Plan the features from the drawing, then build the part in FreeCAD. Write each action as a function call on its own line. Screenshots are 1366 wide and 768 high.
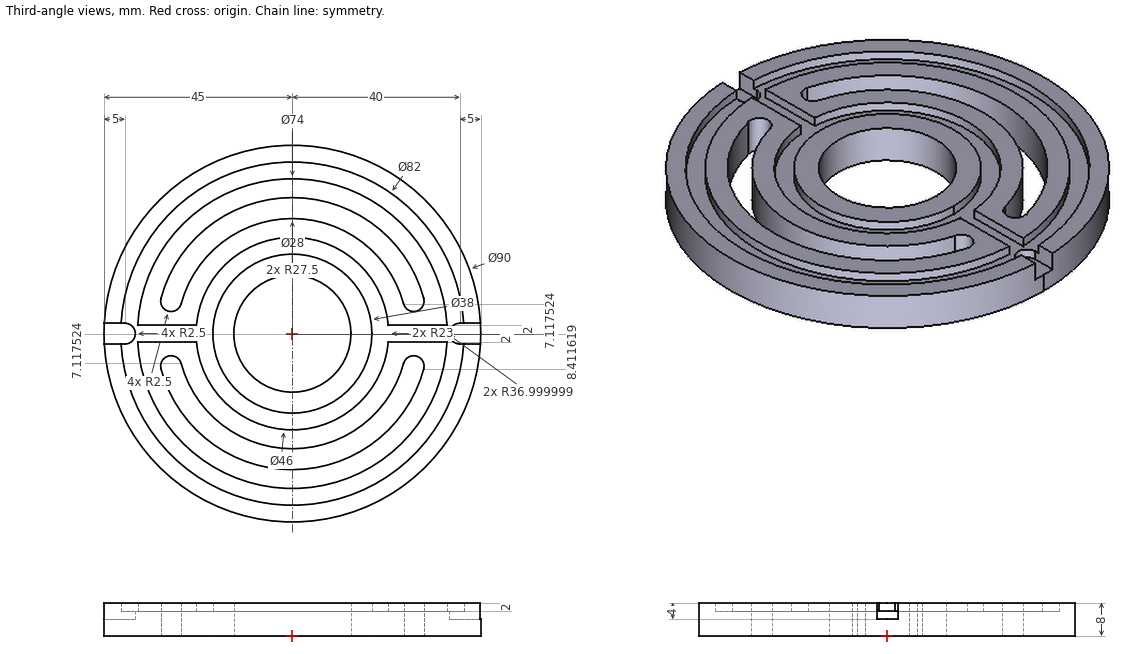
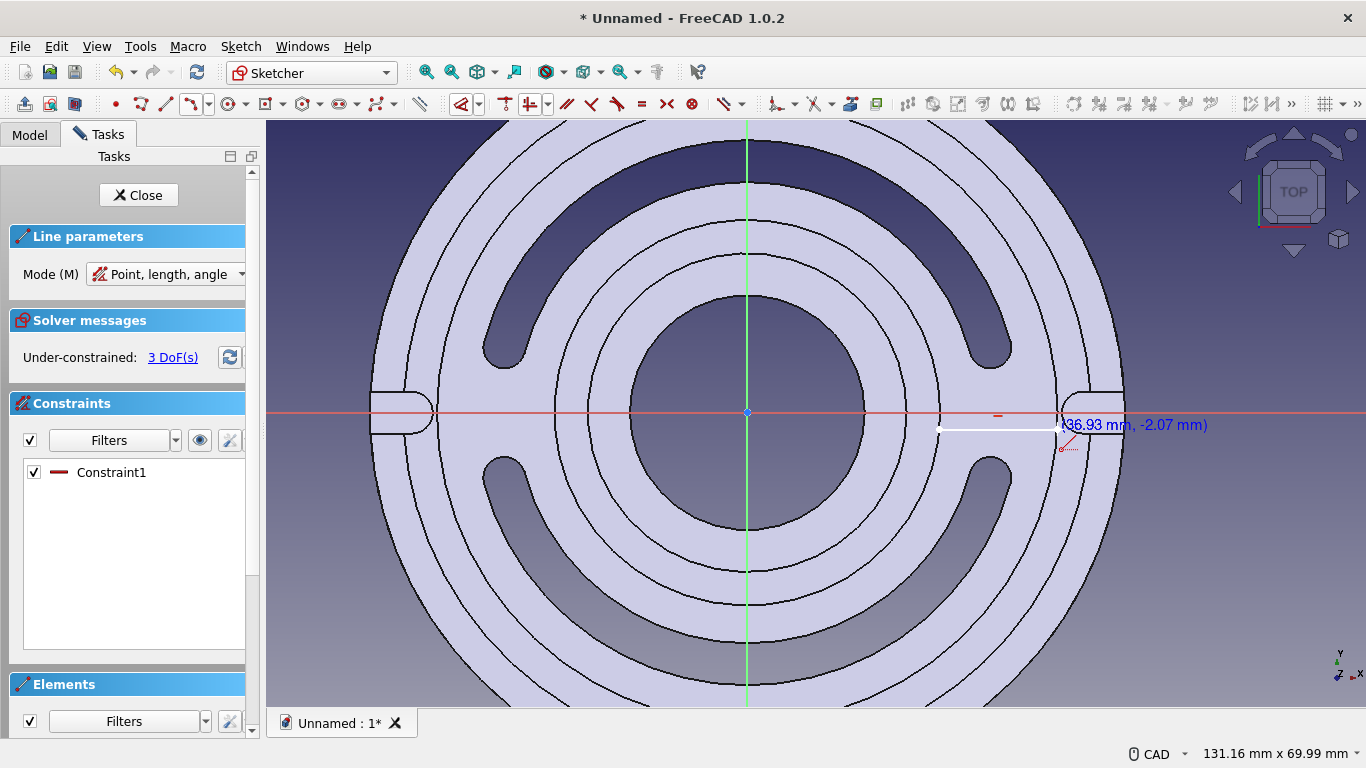
click(1057, 396)
click(939, 396)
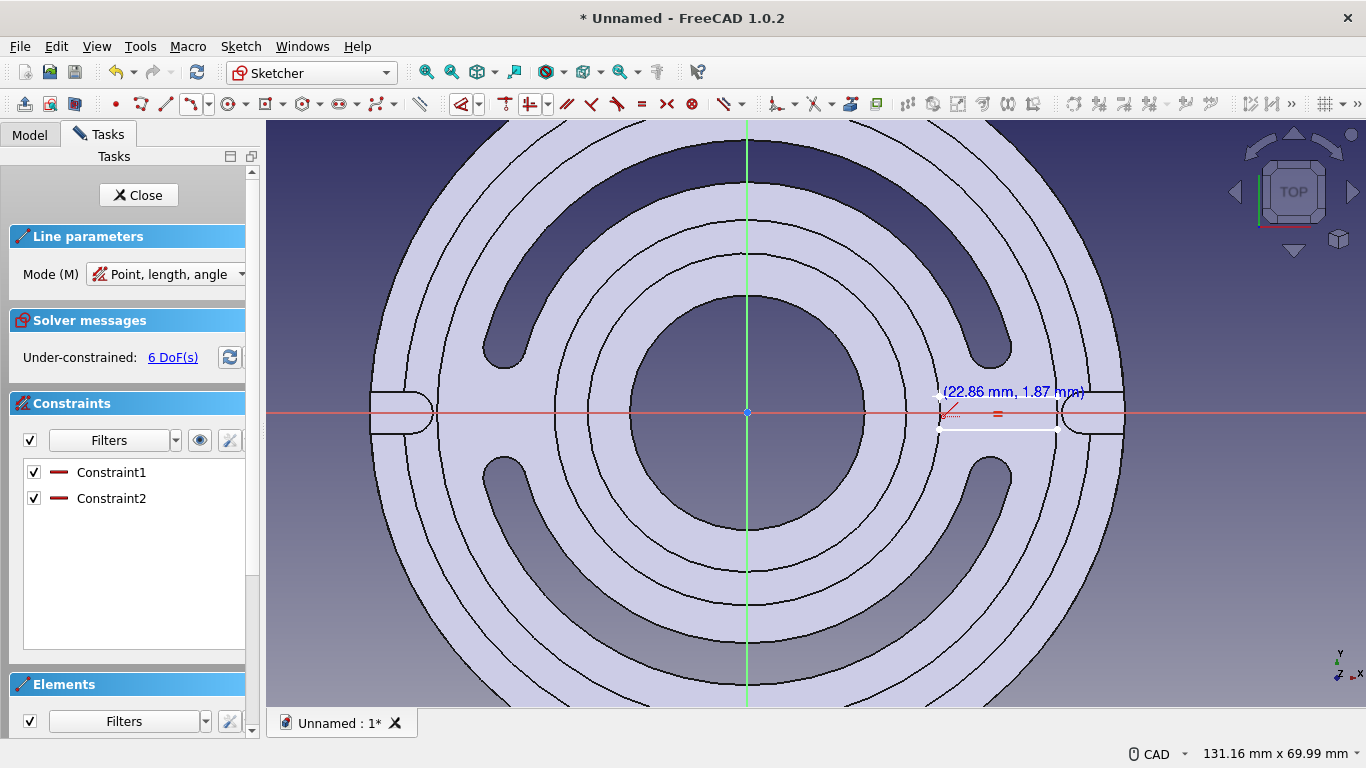
key(g)
key(3)
key(a)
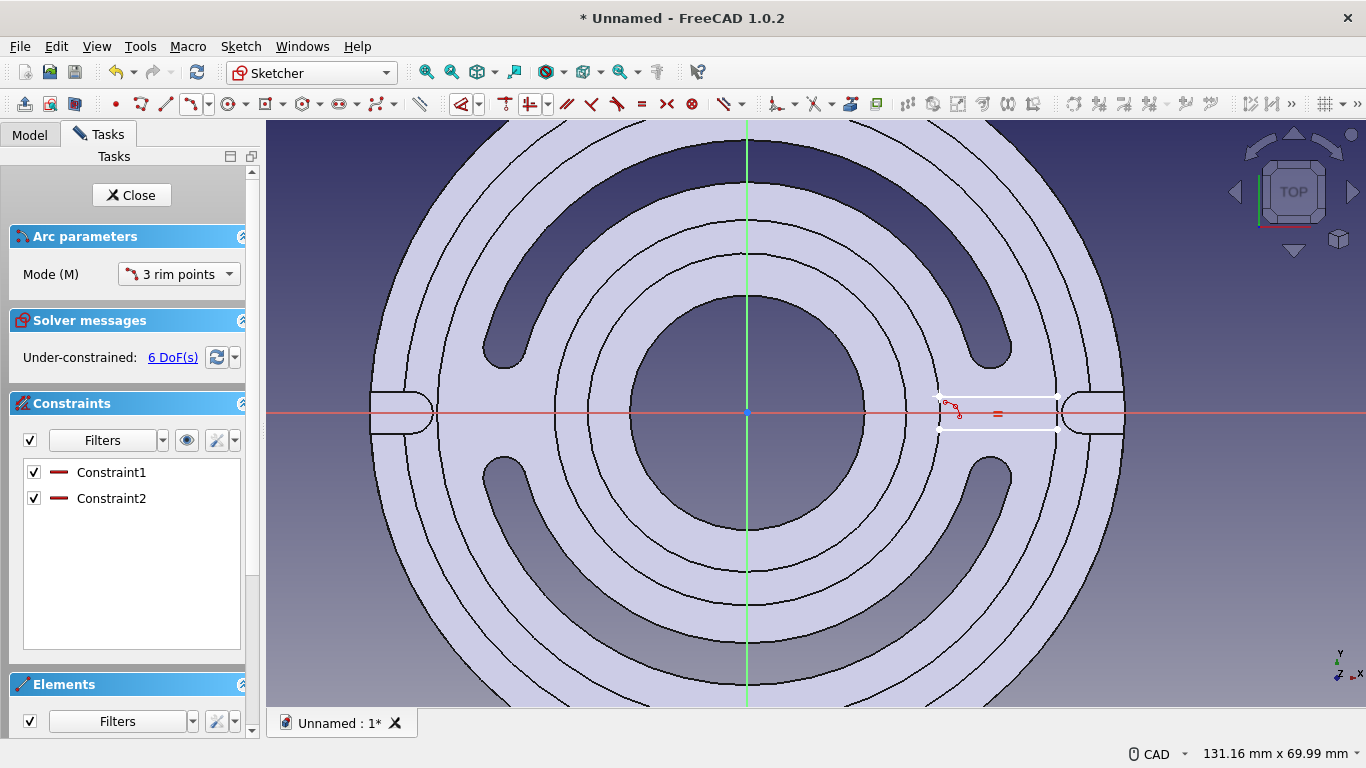
click(1057, 430)
click(1057, 397)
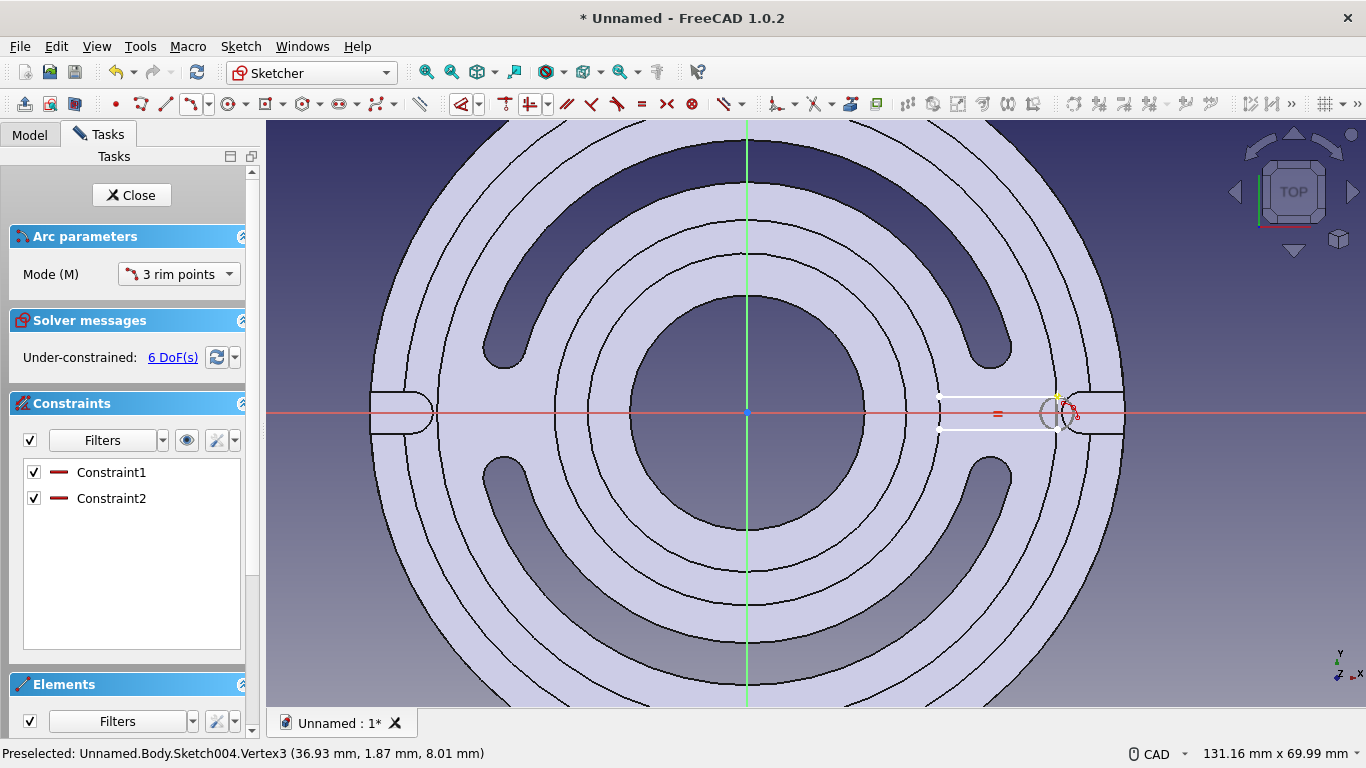
scroll(1058, 416, up, 18)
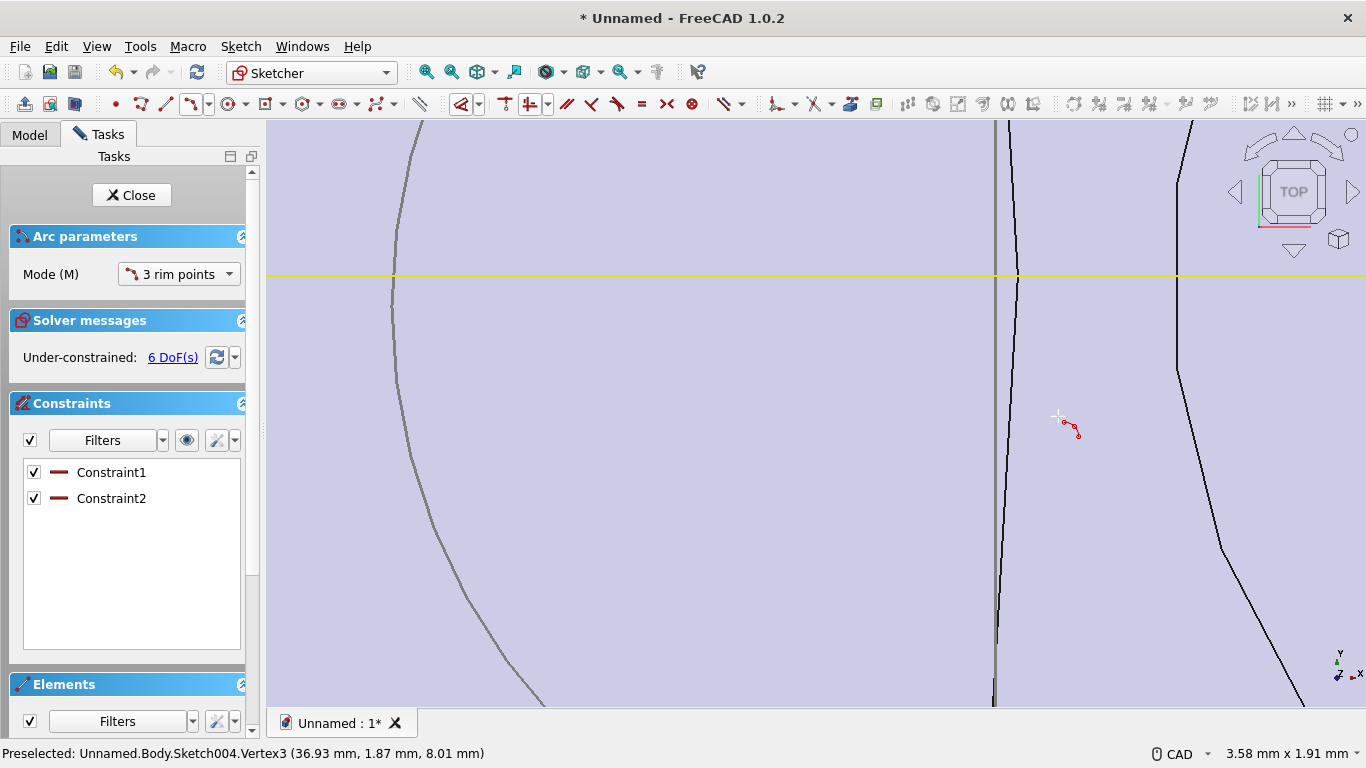
click(1017, 399)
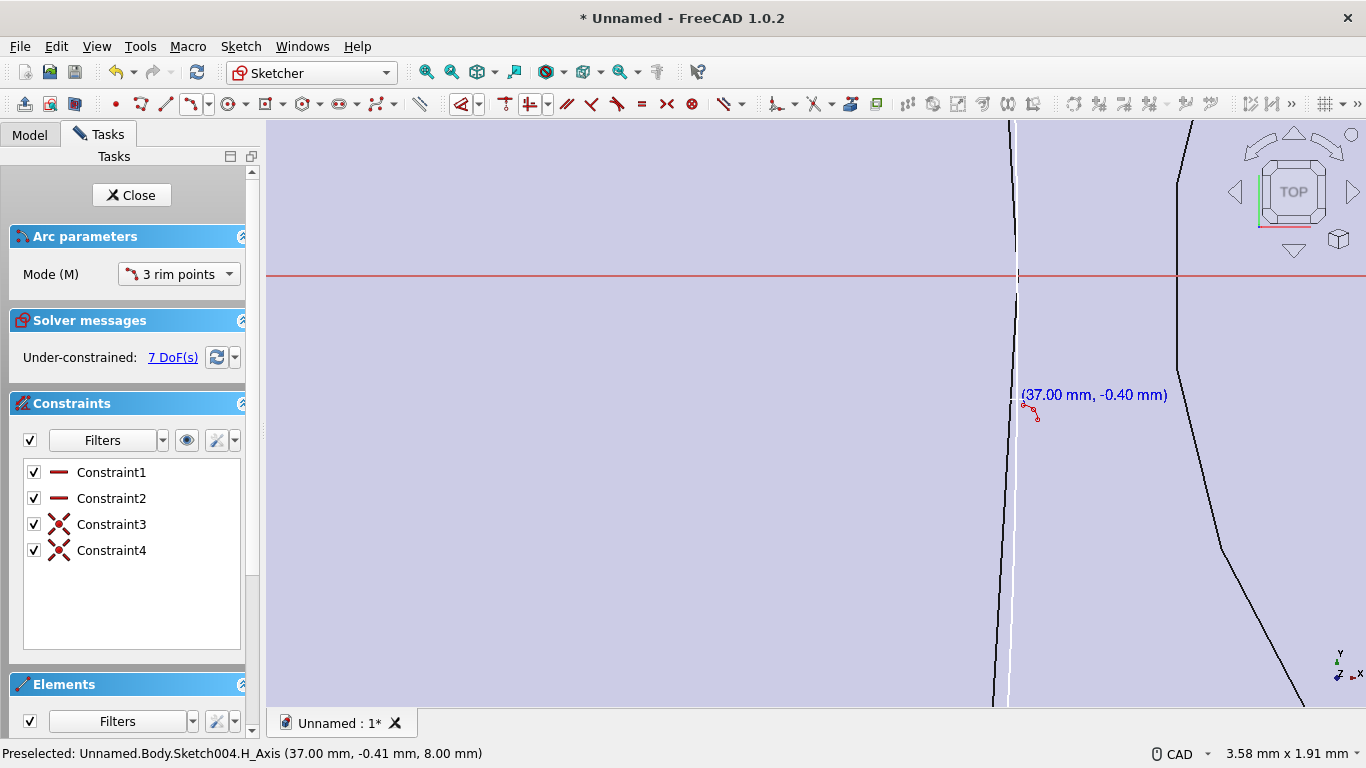
scroll(1130, 418, down, 17)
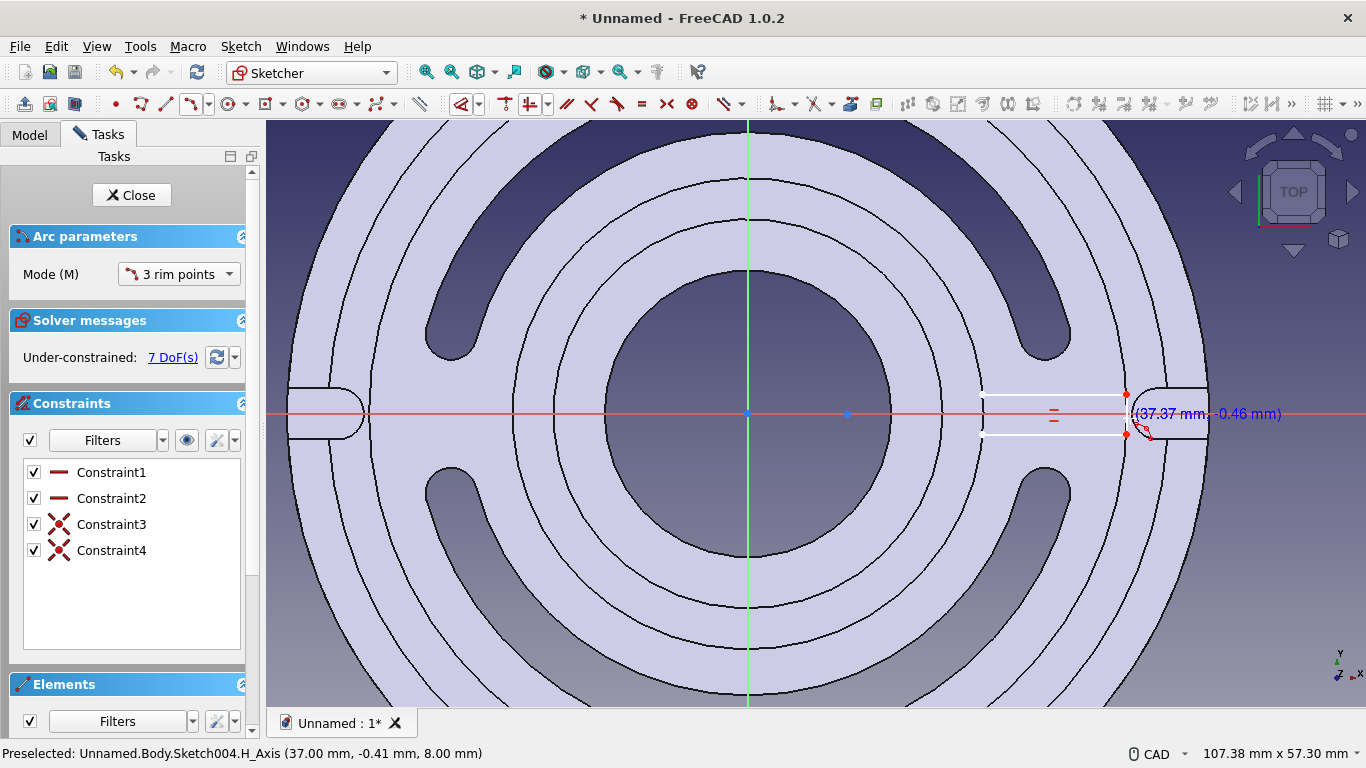
click(982, 395)
click(982, 435)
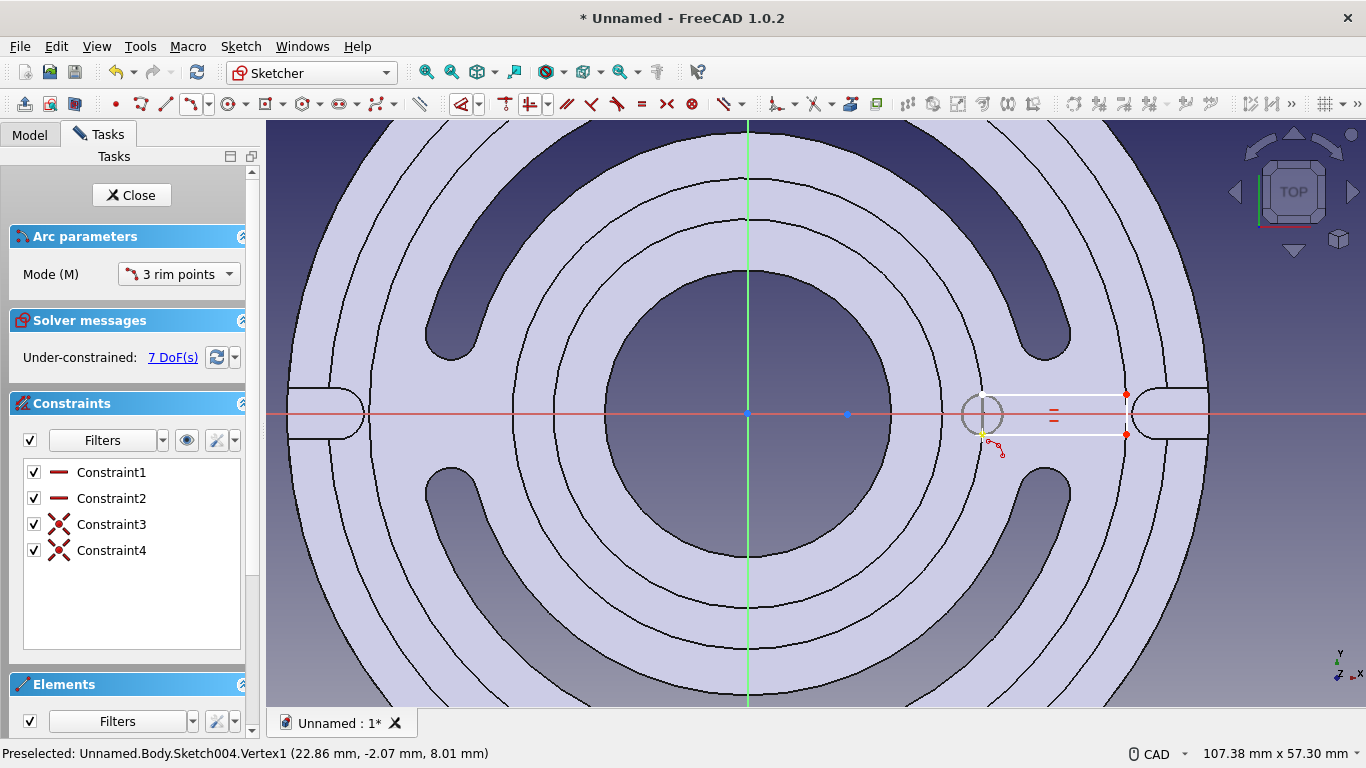
scroll(984, 418, up, 15)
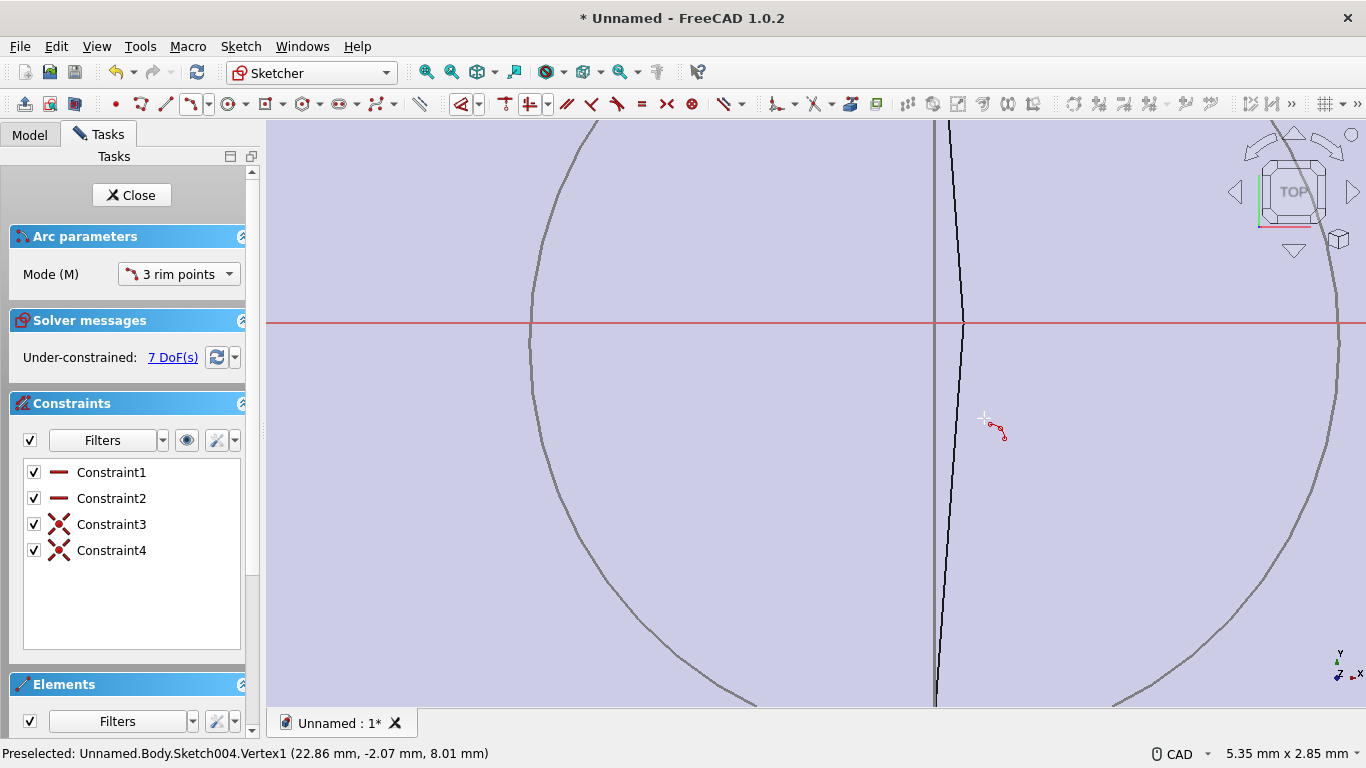
click(963, 406)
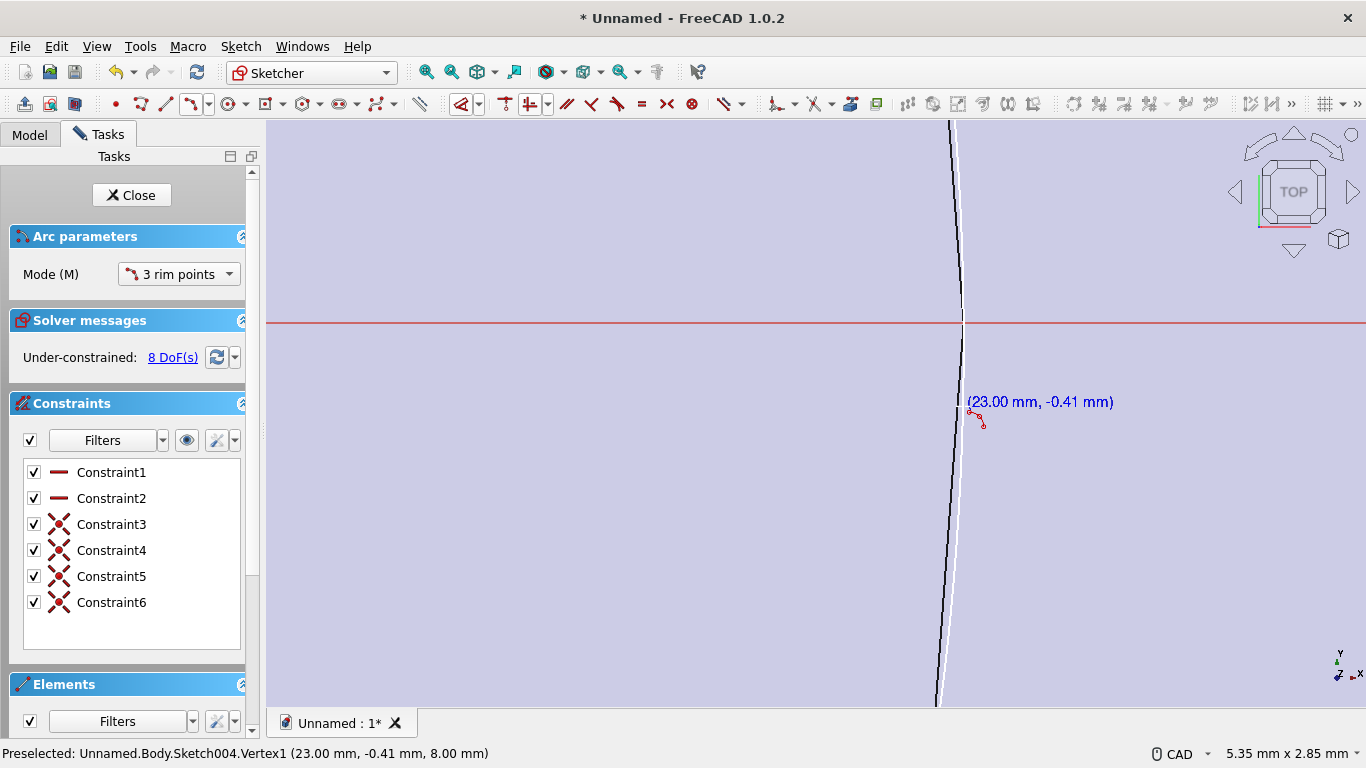
key(g)
key(l)